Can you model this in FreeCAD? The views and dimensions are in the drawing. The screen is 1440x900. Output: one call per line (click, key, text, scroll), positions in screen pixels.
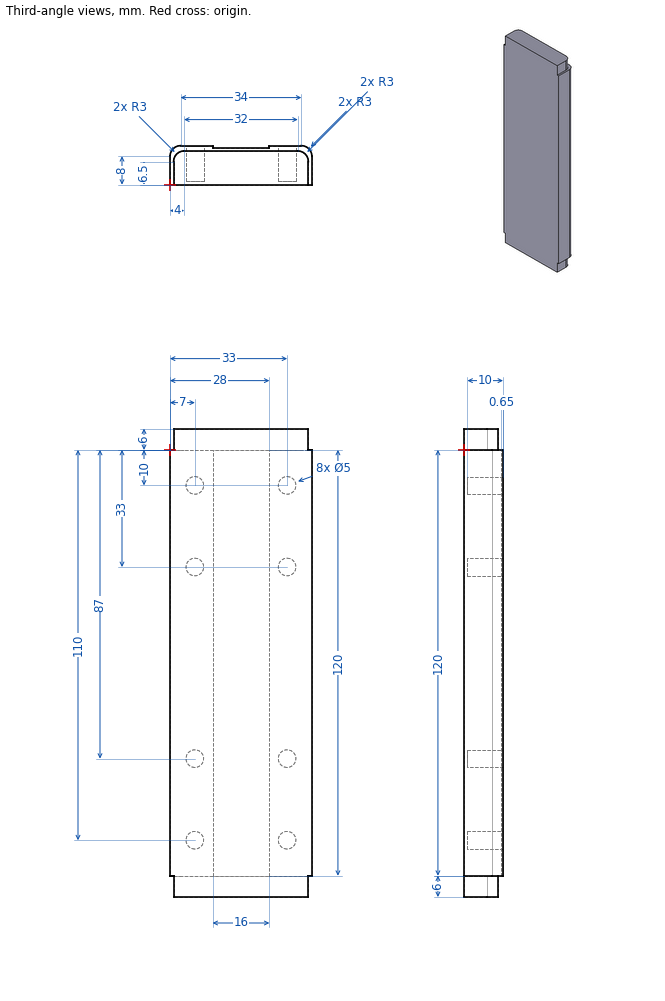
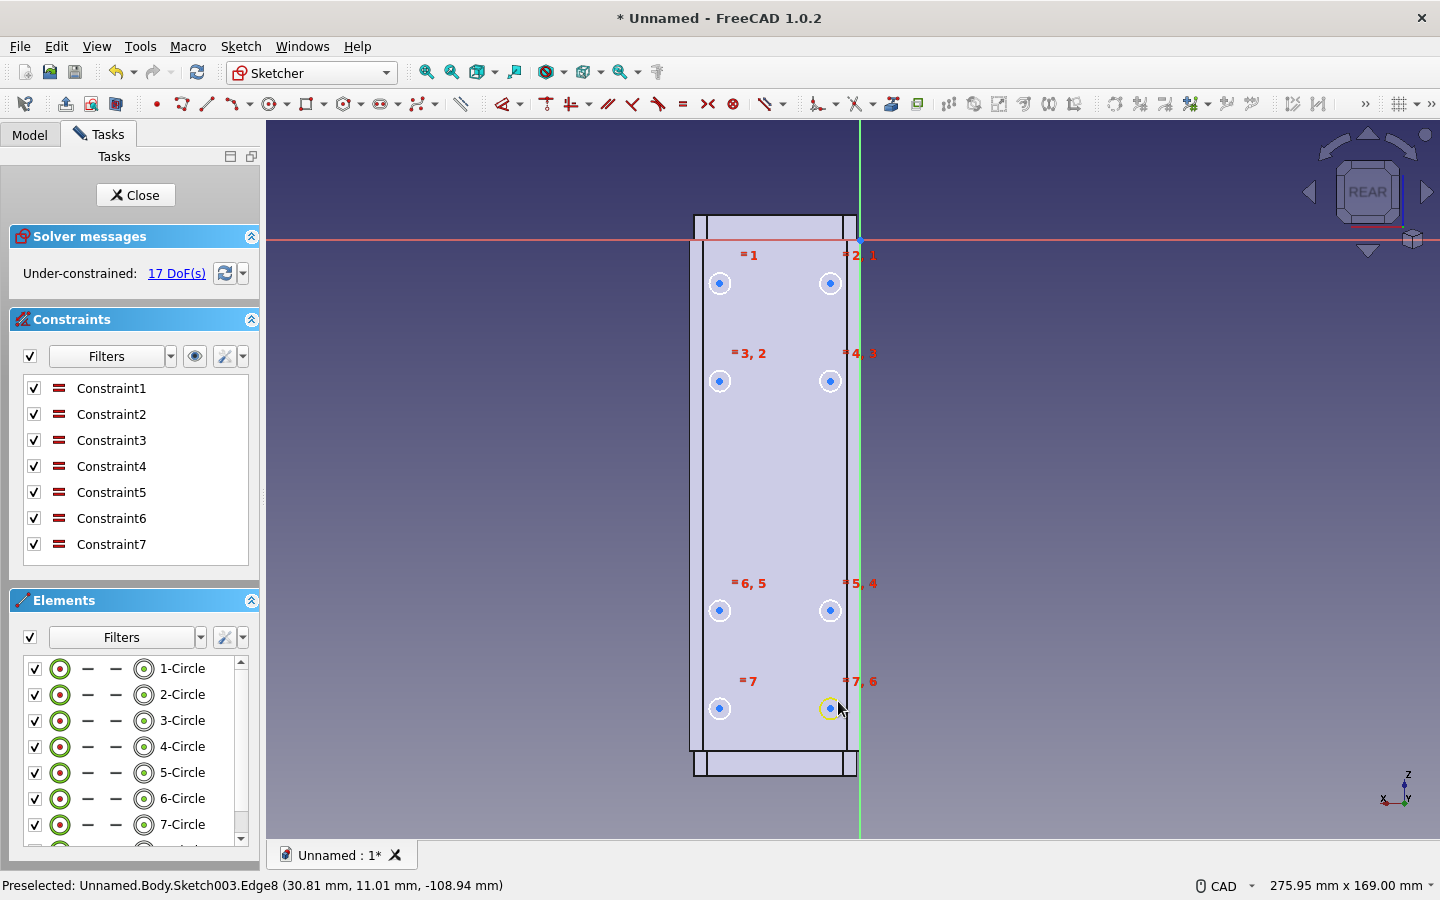
click(720, 284)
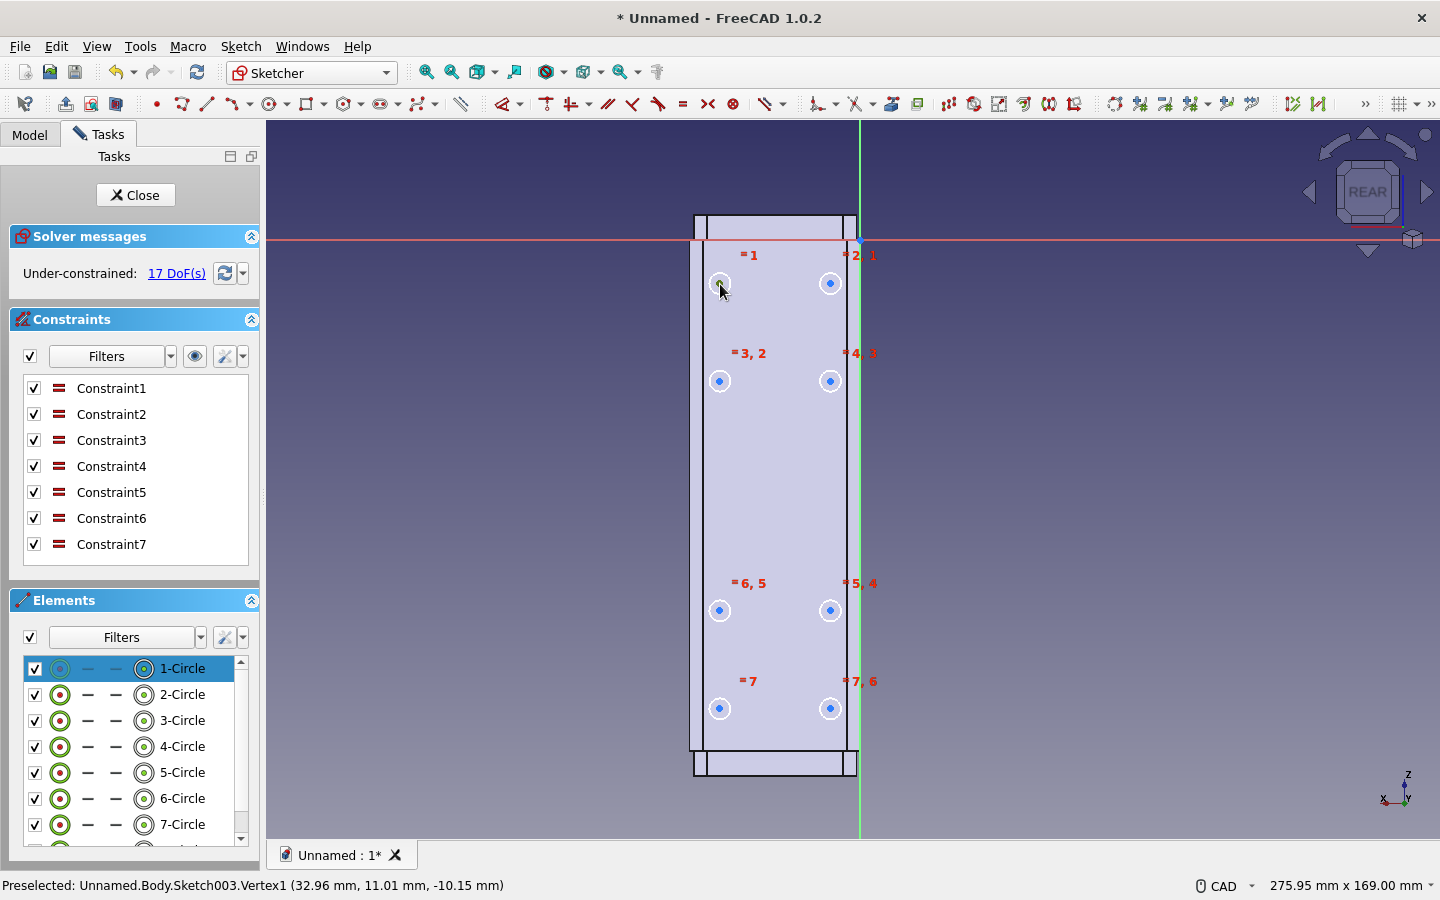
click(831, 284)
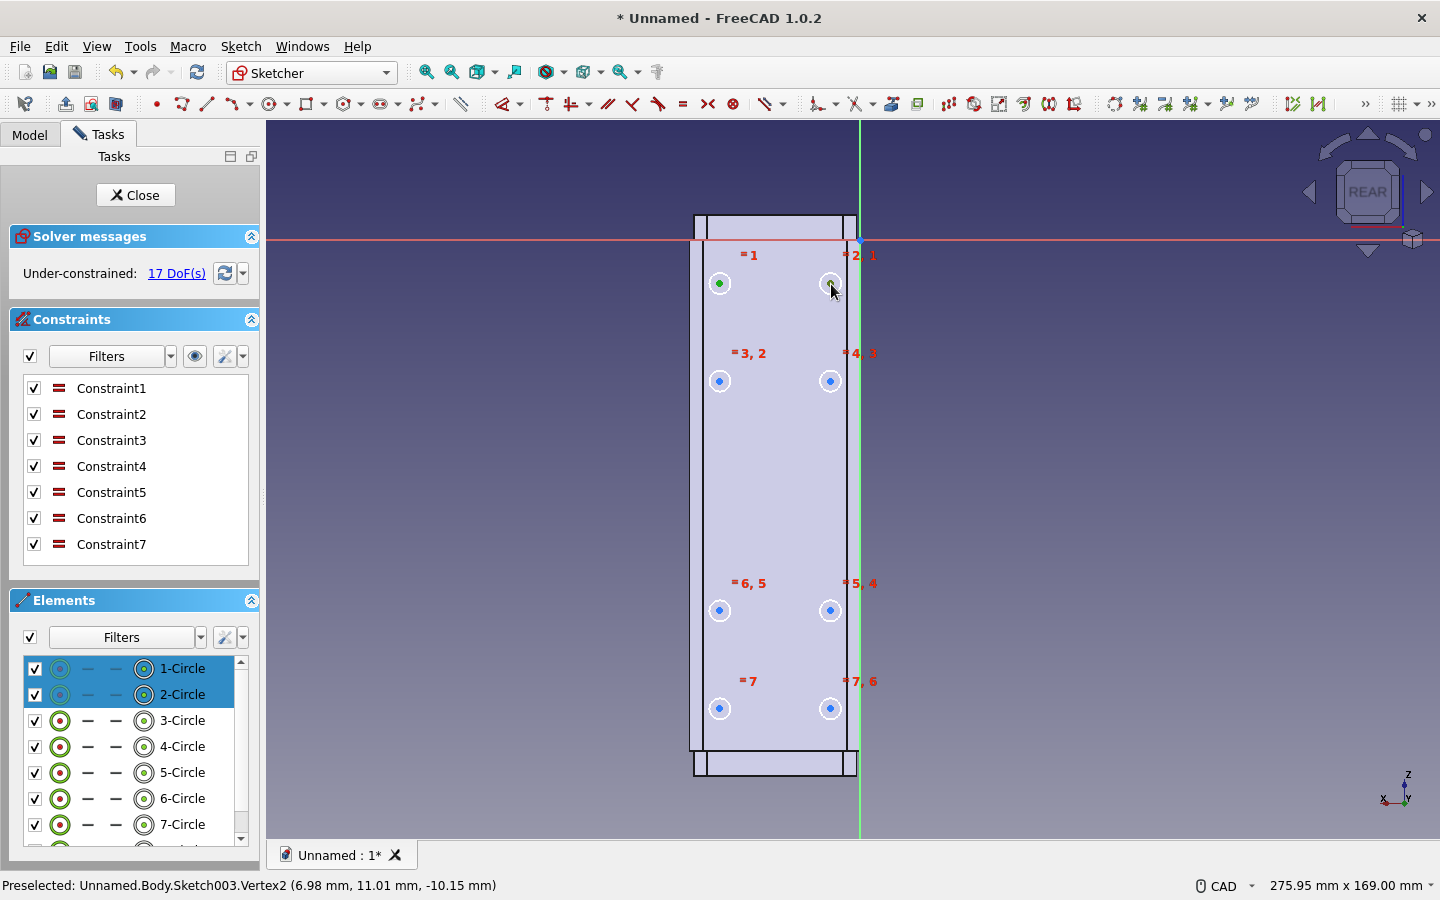
key(h)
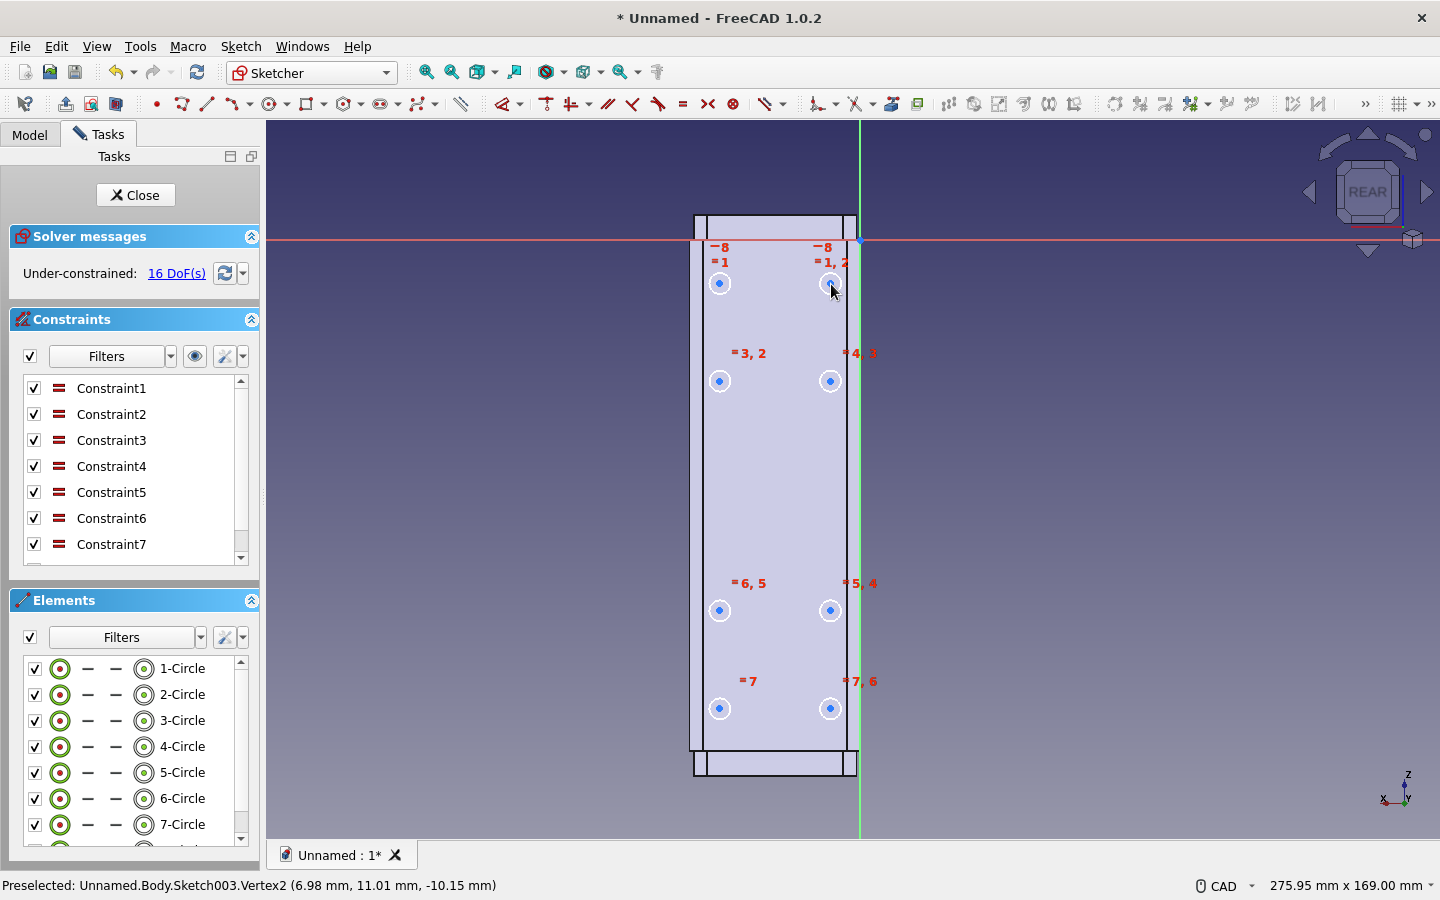
click(720, 284)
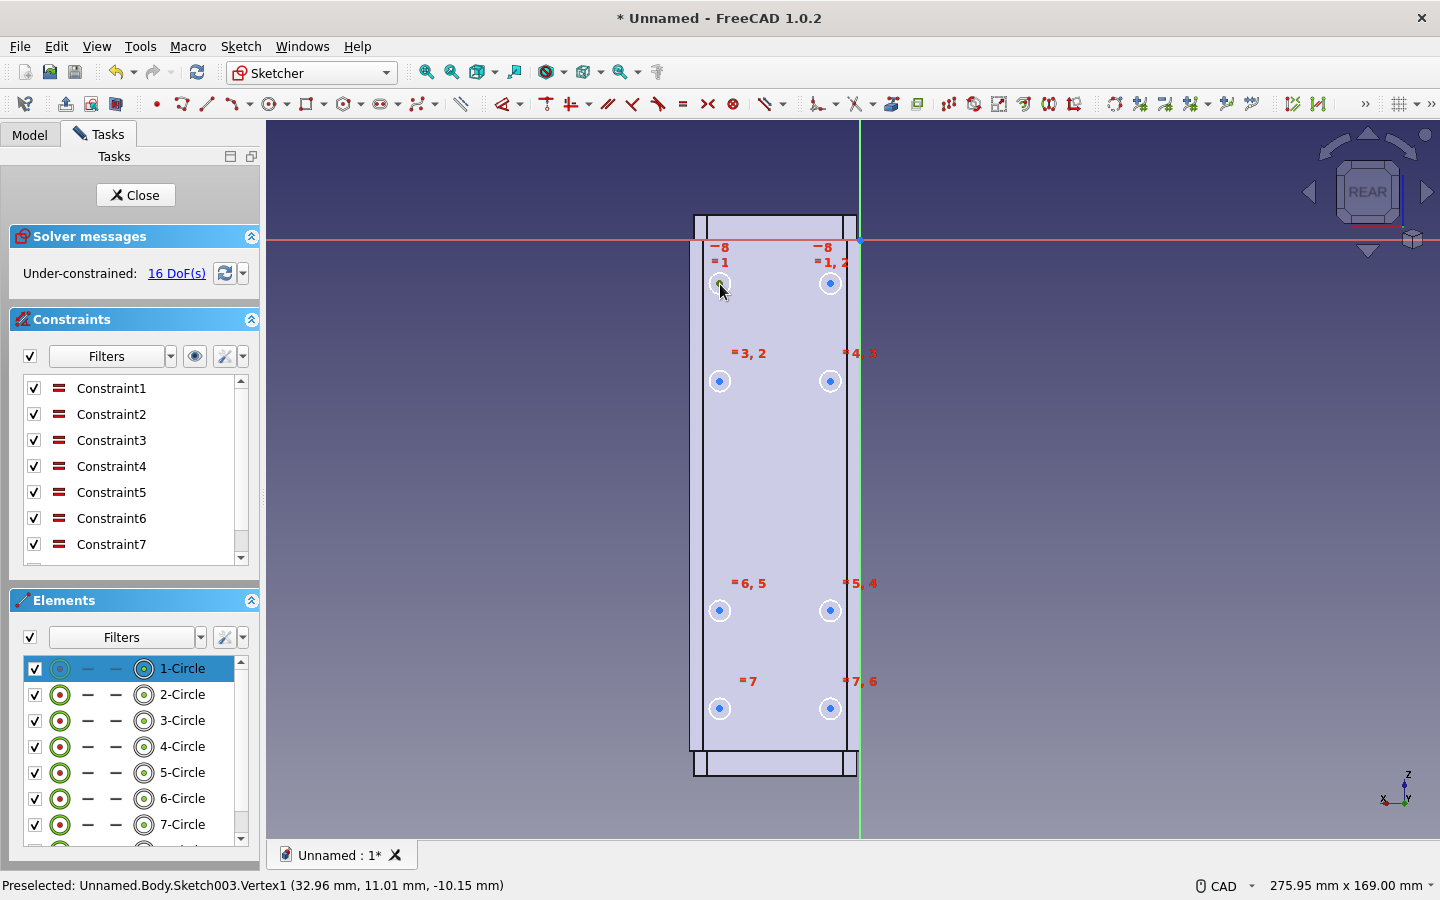
click(720, 381)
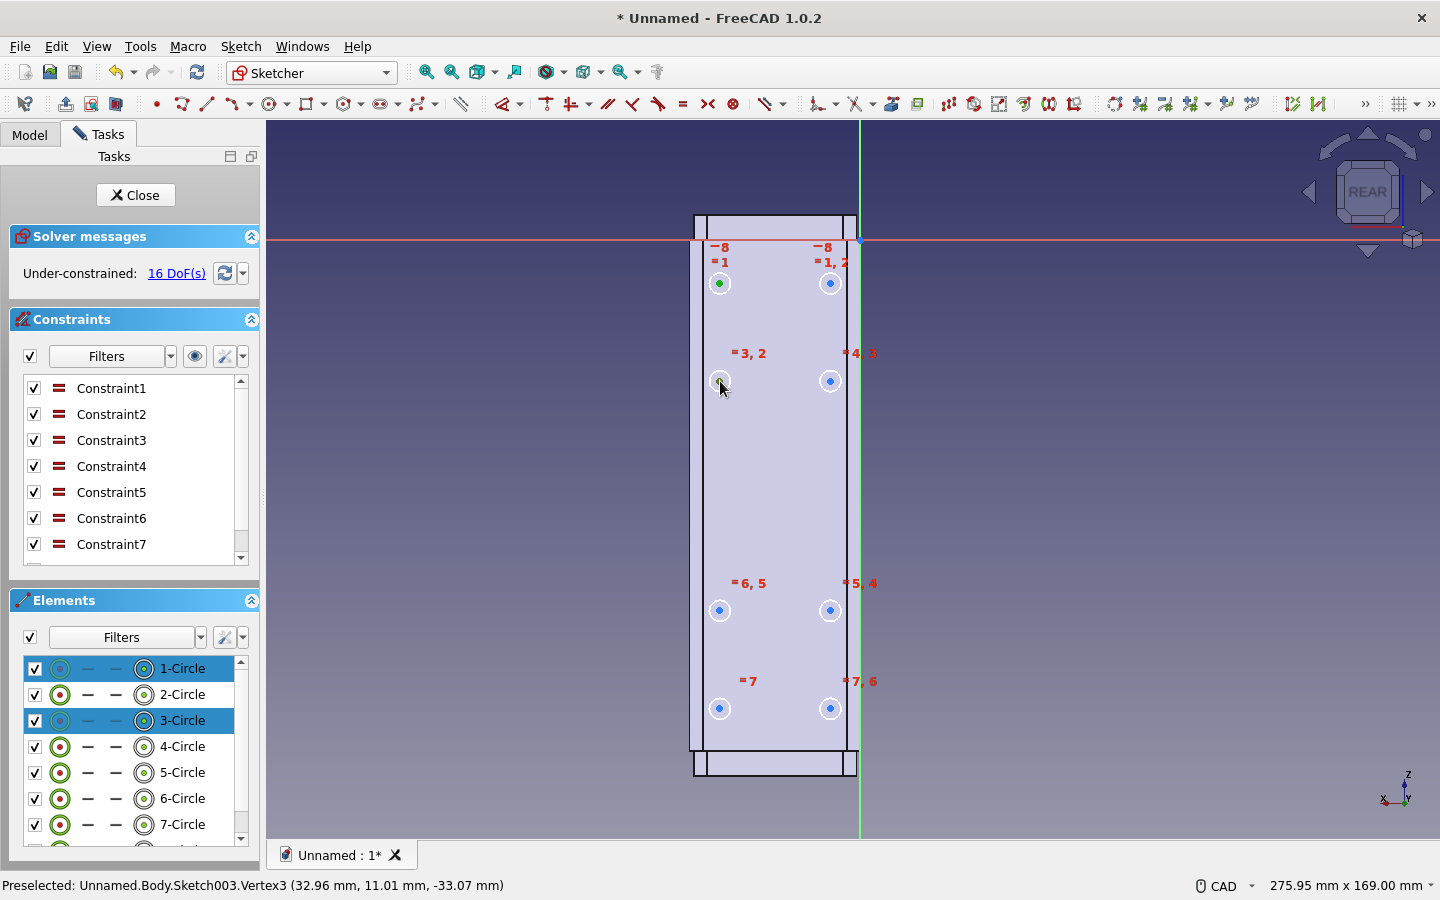
click(588, 104)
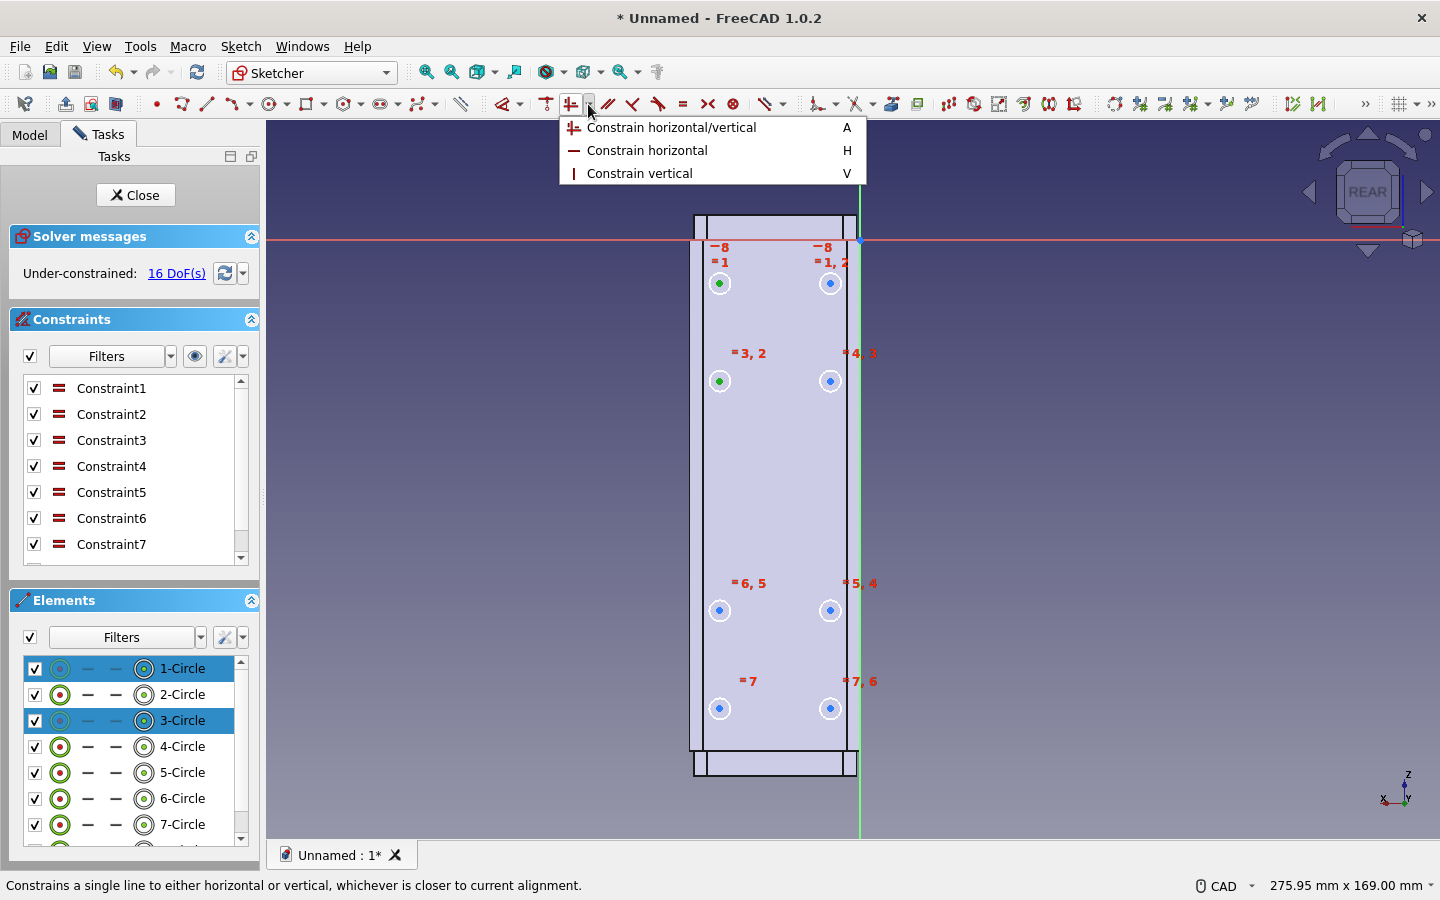
click(713, 174)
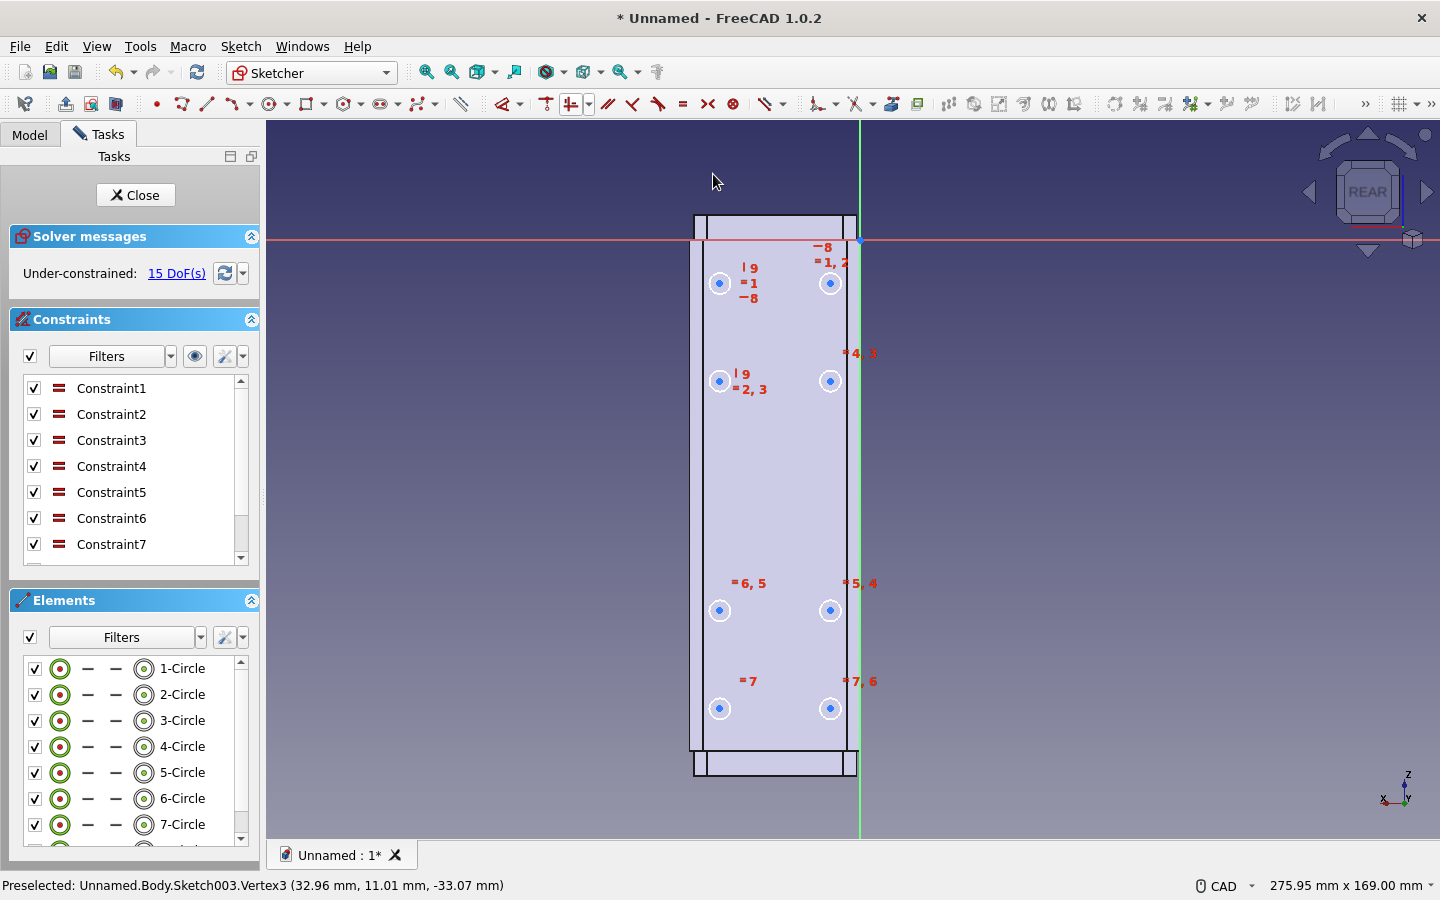
click(831, 284)